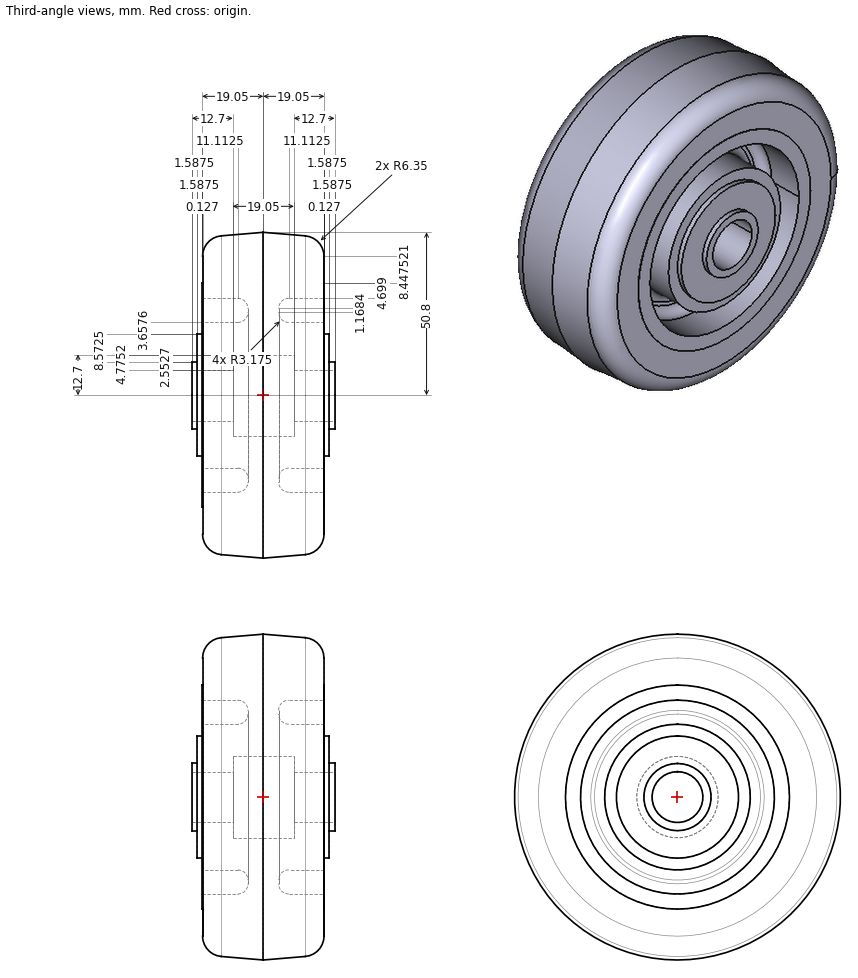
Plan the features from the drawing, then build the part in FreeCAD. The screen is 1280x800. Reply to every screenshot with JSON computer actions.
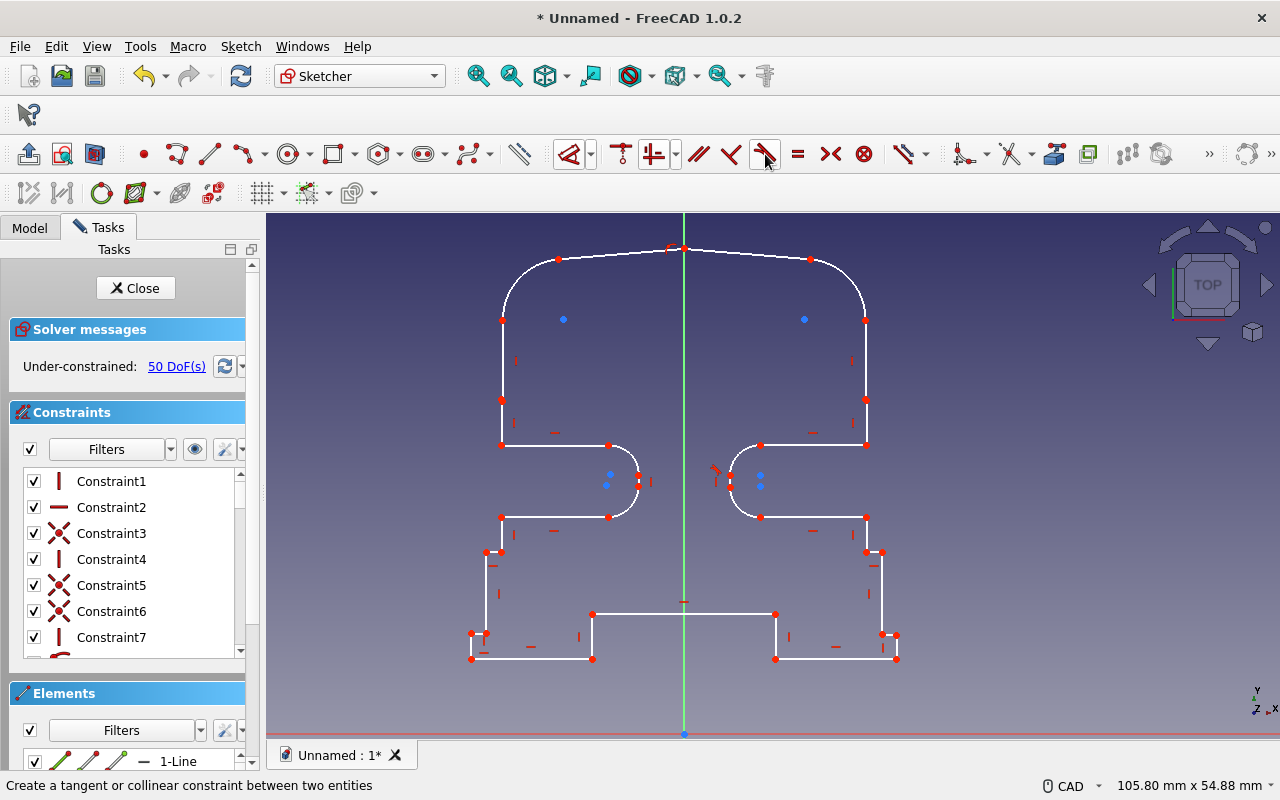
{"action": "scroll", "coordinate": [730, 482], "scroll_direction": "up", "scroll_amount": 5}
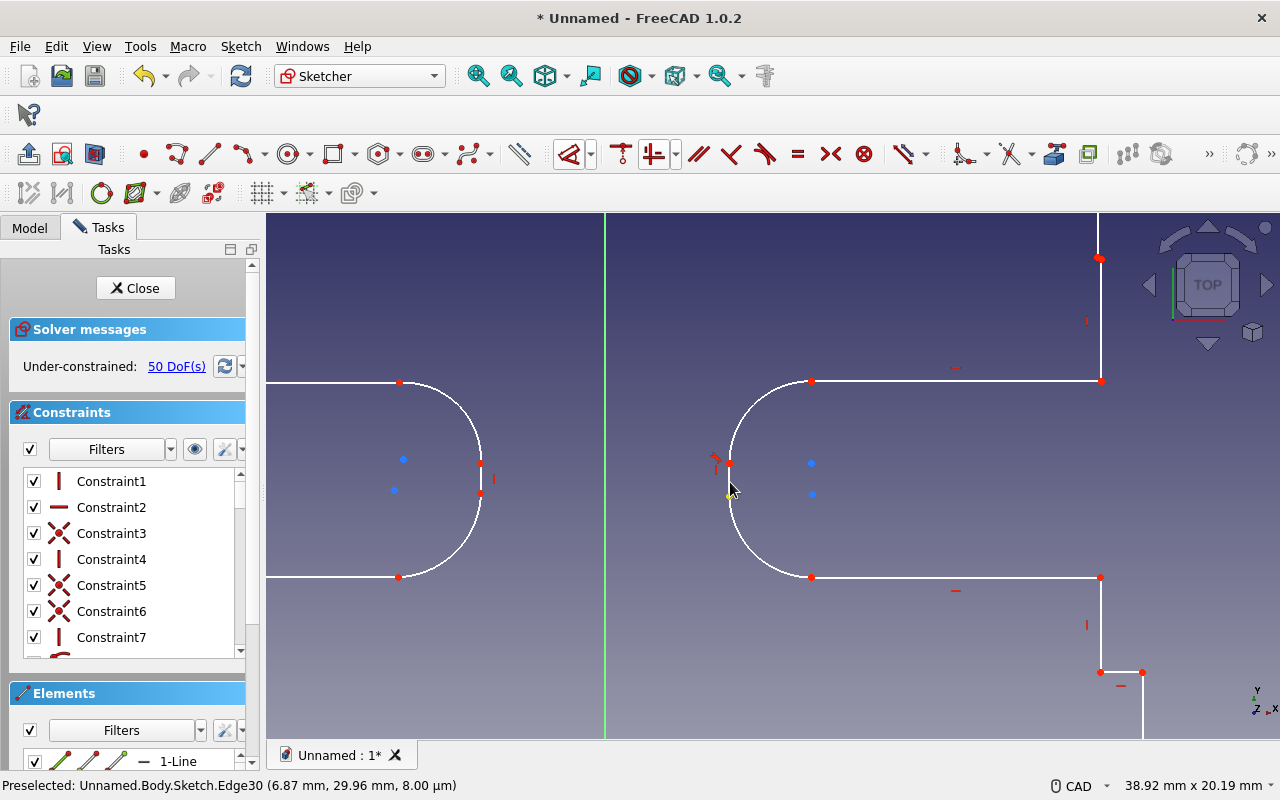
{"action": "left_click", "coordinate": [729, 480]}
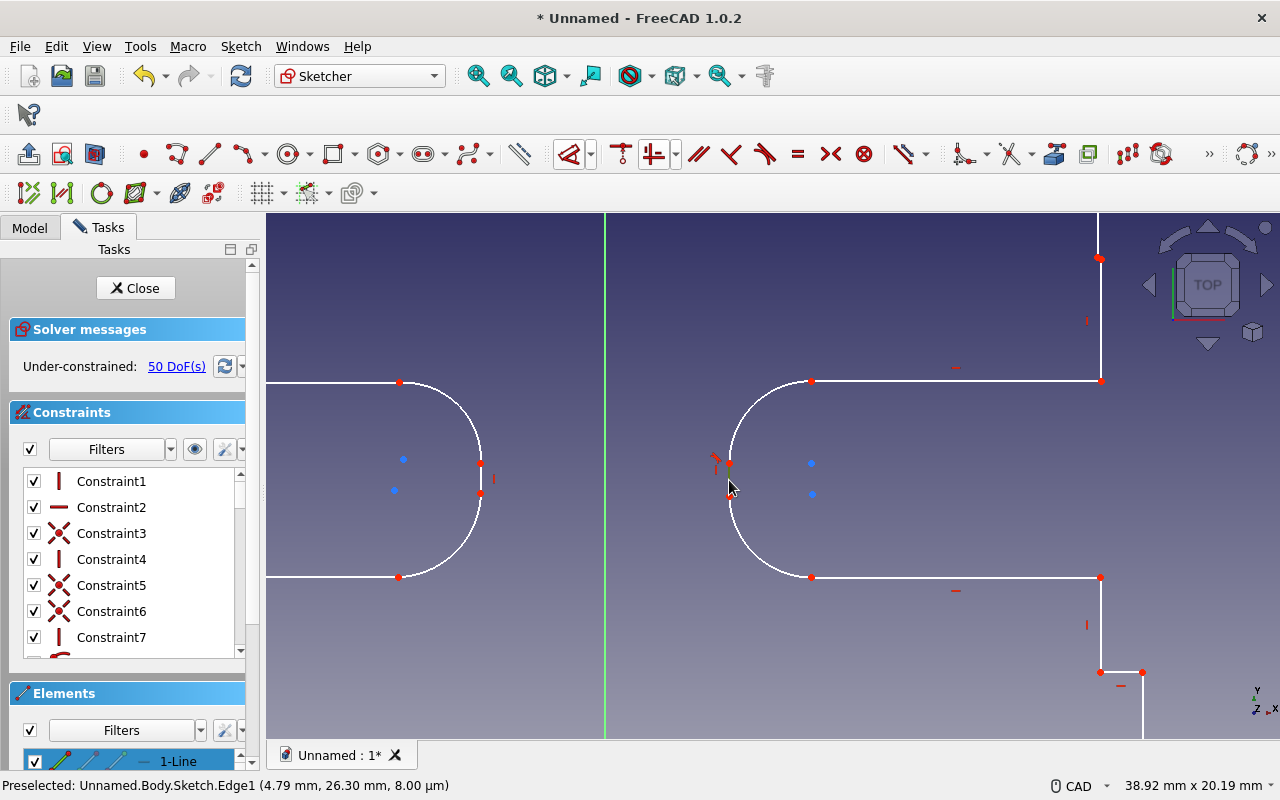
{"action": "left_click", "coordinate": [739, 533]}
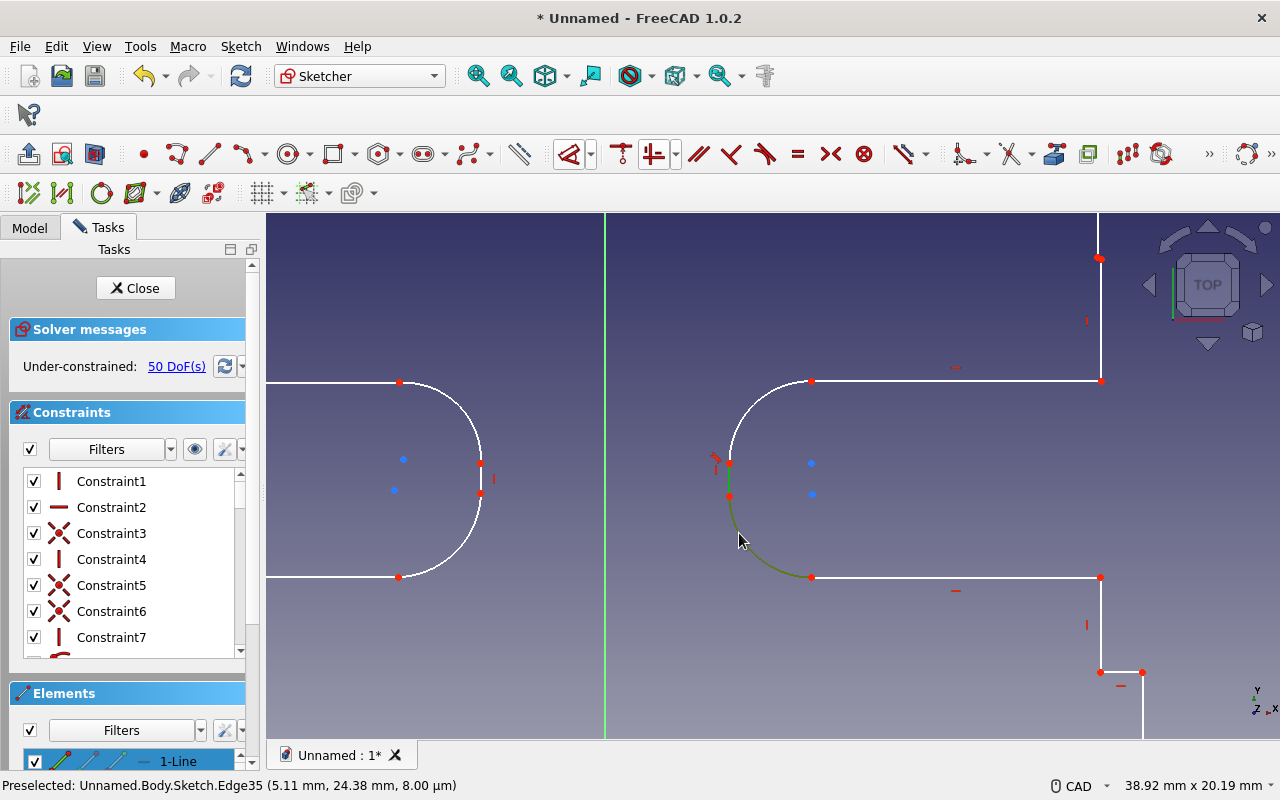
{"action": "left_click", "coordinate": [765, 154]}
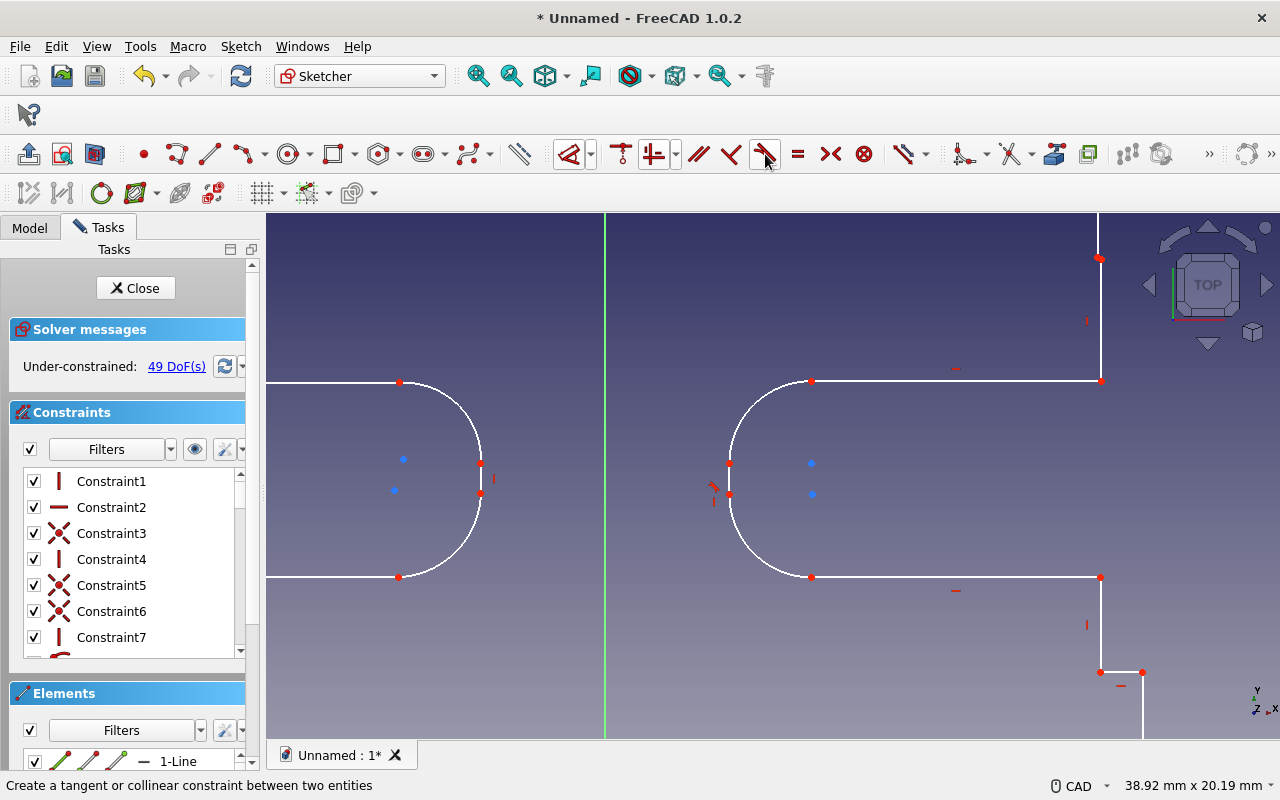
{"action": "scroll", "coordinate": [737, 467], "scroll_direction": "down", "scroll_amount": 7}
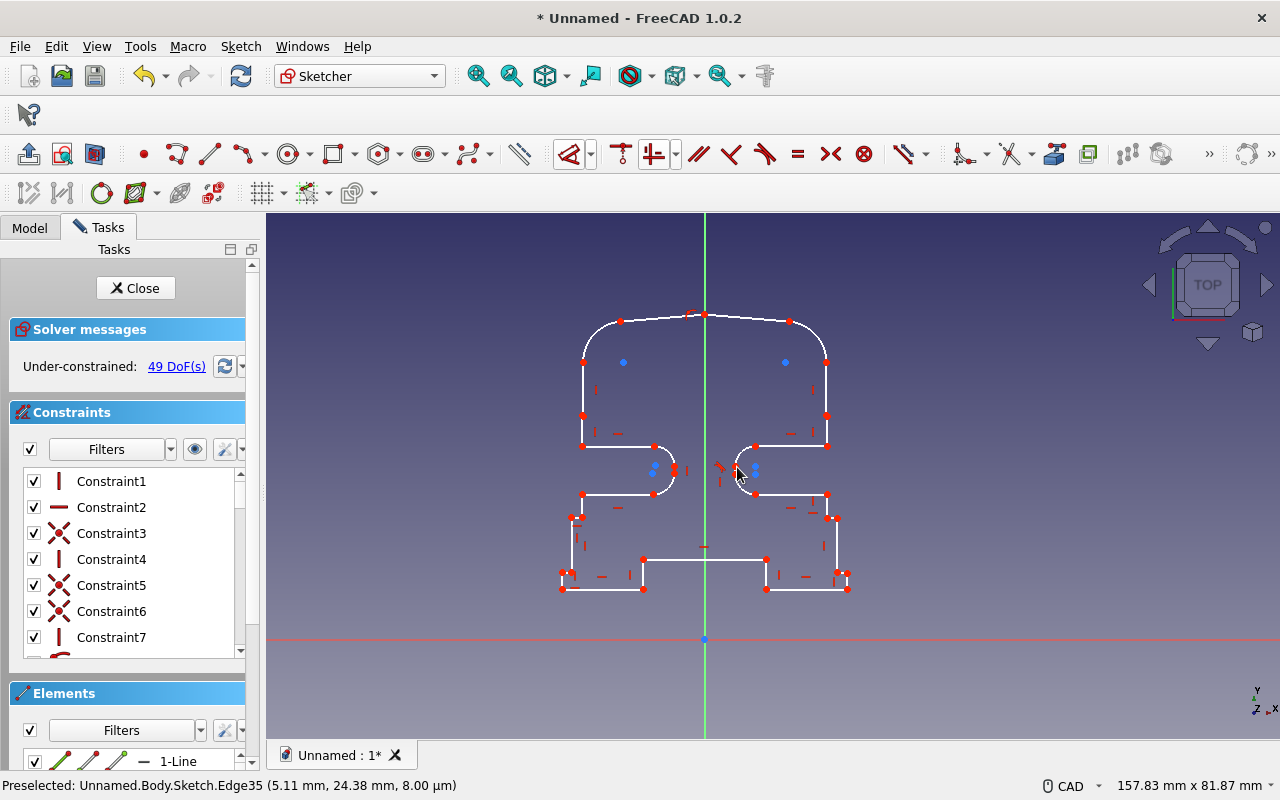
{"action": "left_click", "coordinate": [777, 446]}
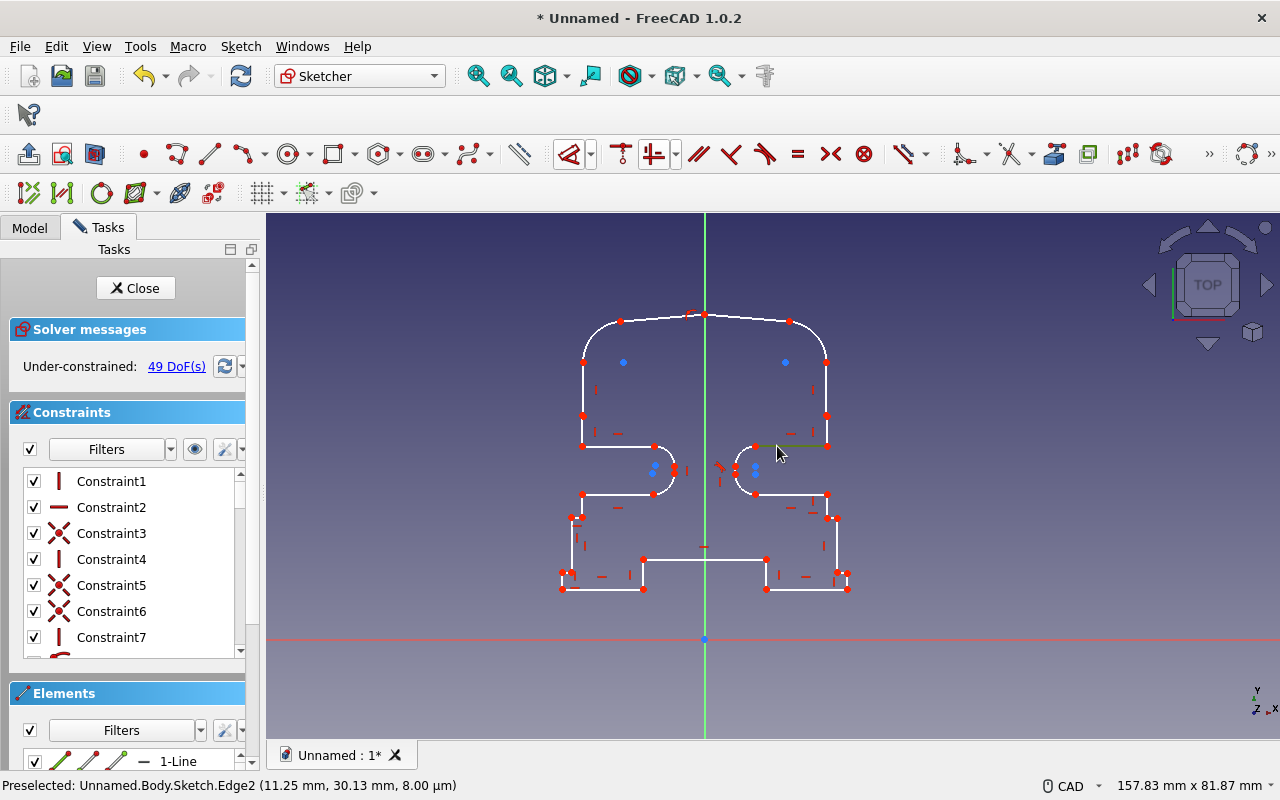
{"action": "scroll", "coordinate": [747, 448], "scroll_direction": "up", "scroll_amount": 2}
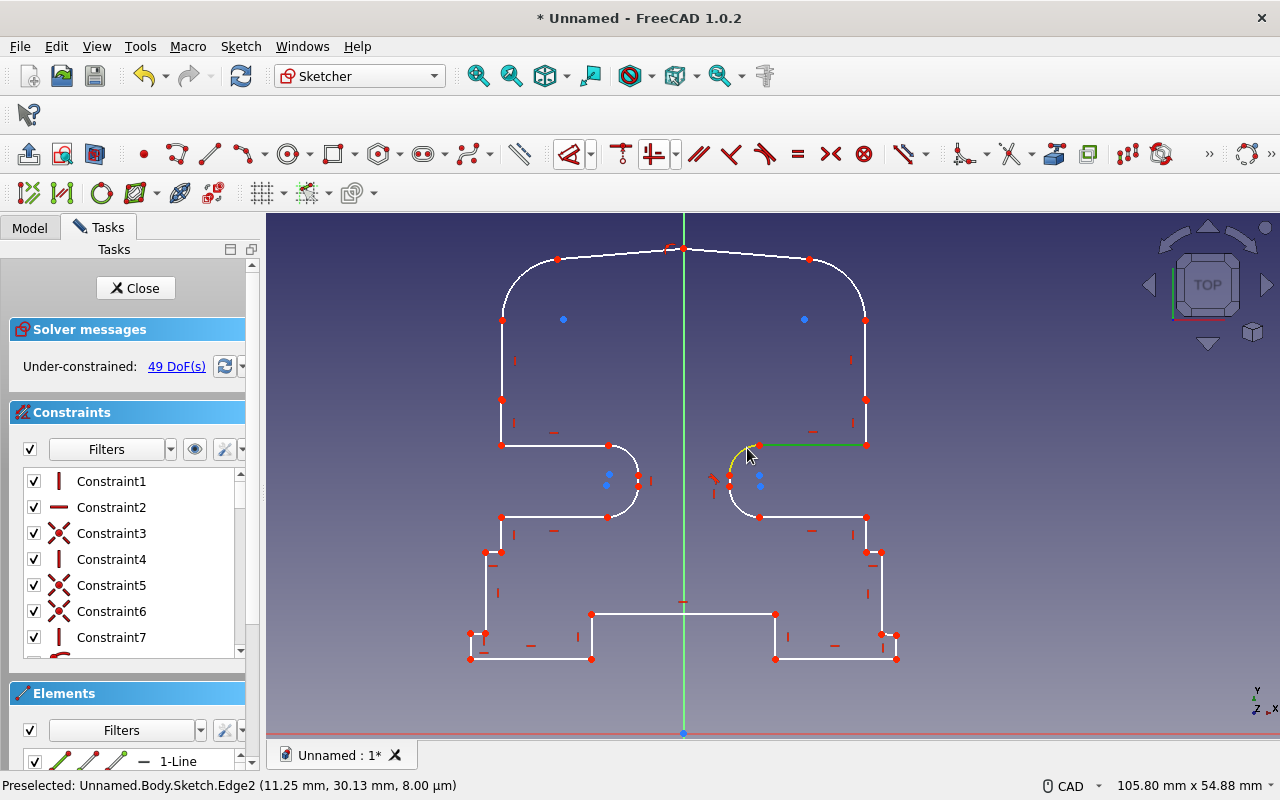
{"action": "left_click", "coordinate": [746, 448]}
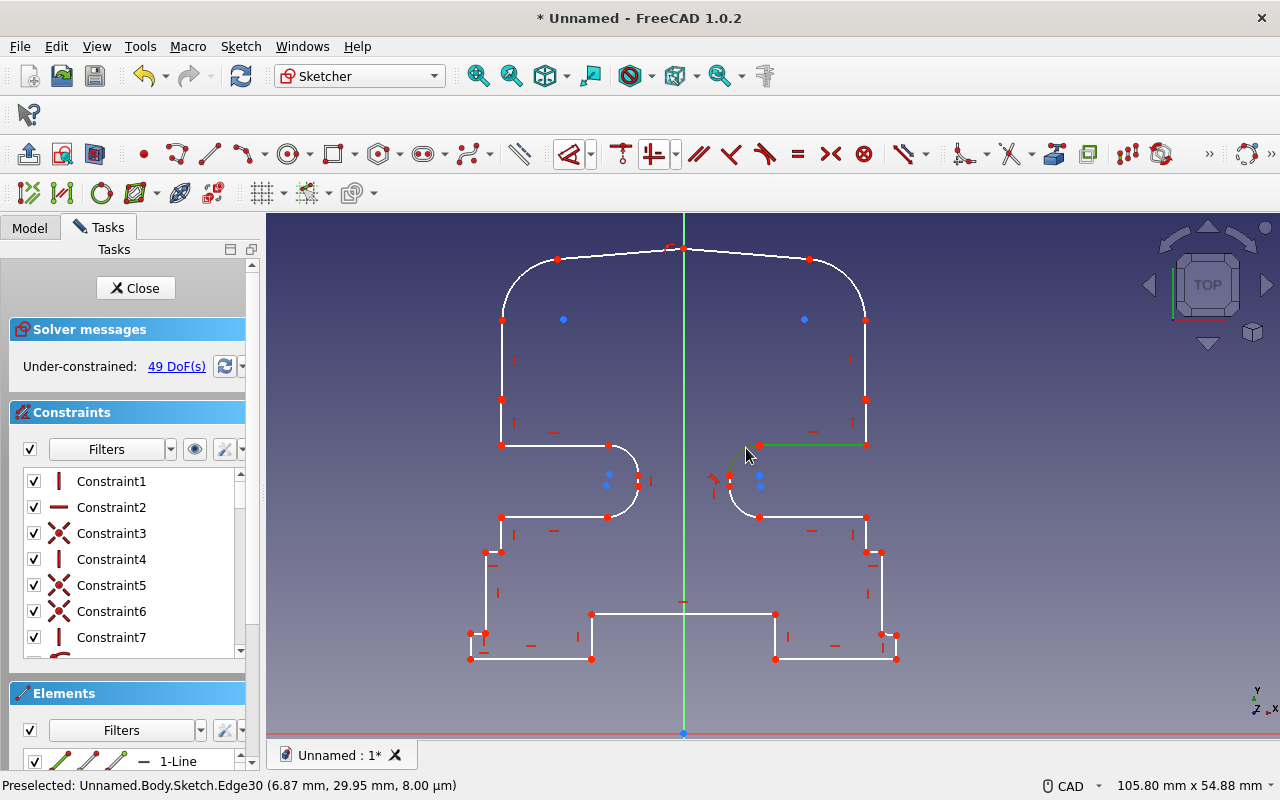
{"action": "left_click", "coordinate": [765, 154]}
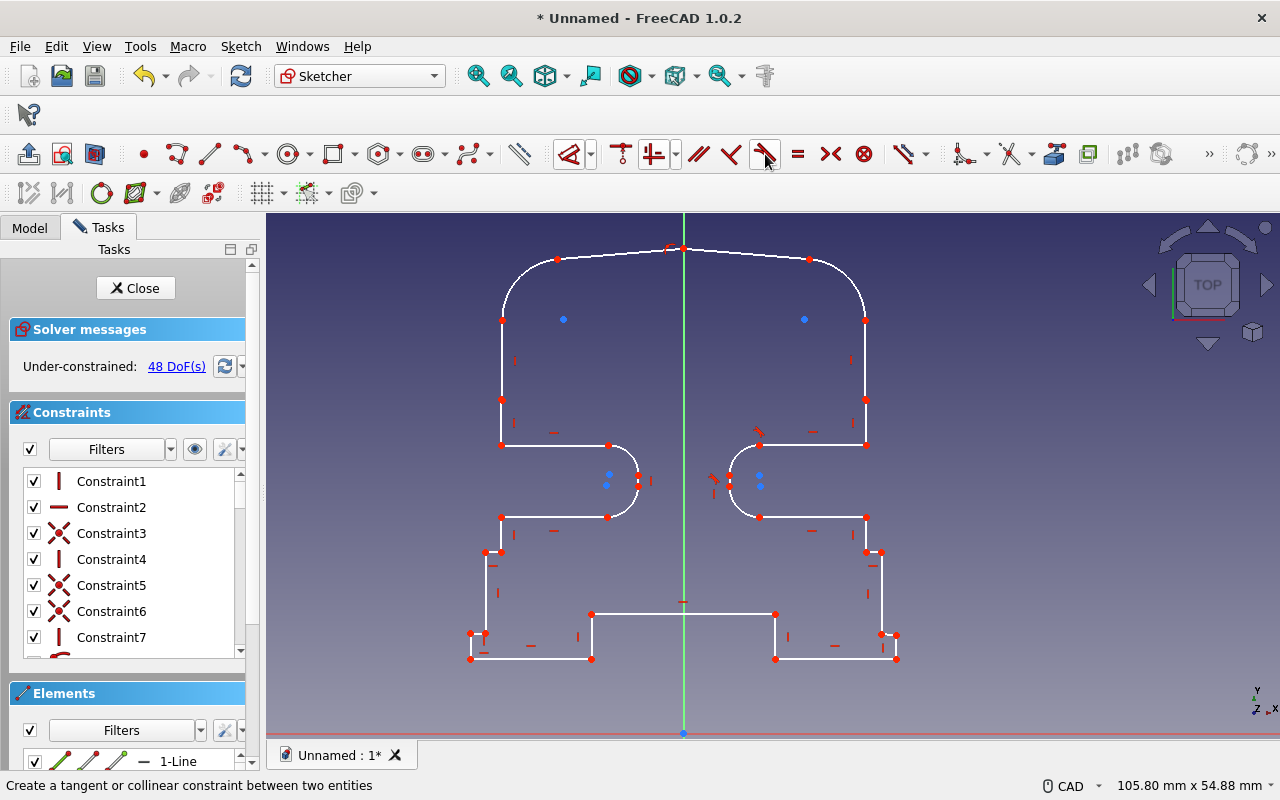
{"action": "left_click", "coordinate": [865, 376]}